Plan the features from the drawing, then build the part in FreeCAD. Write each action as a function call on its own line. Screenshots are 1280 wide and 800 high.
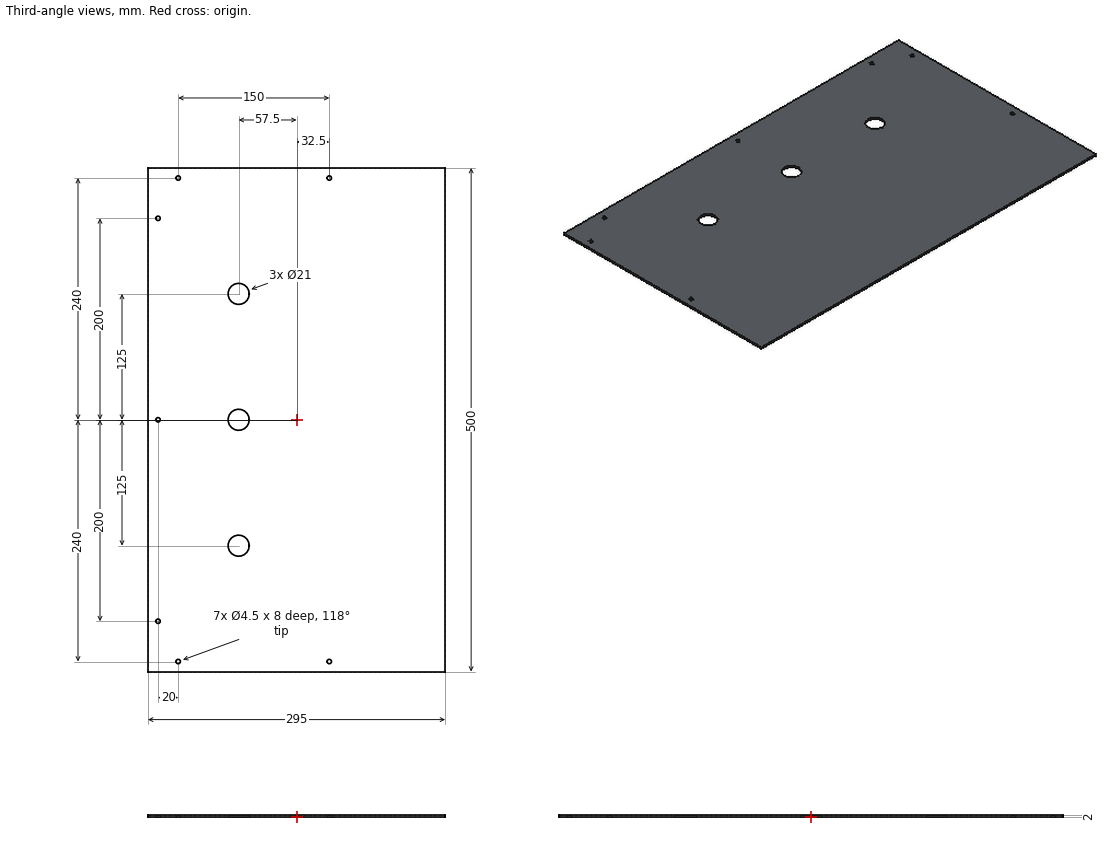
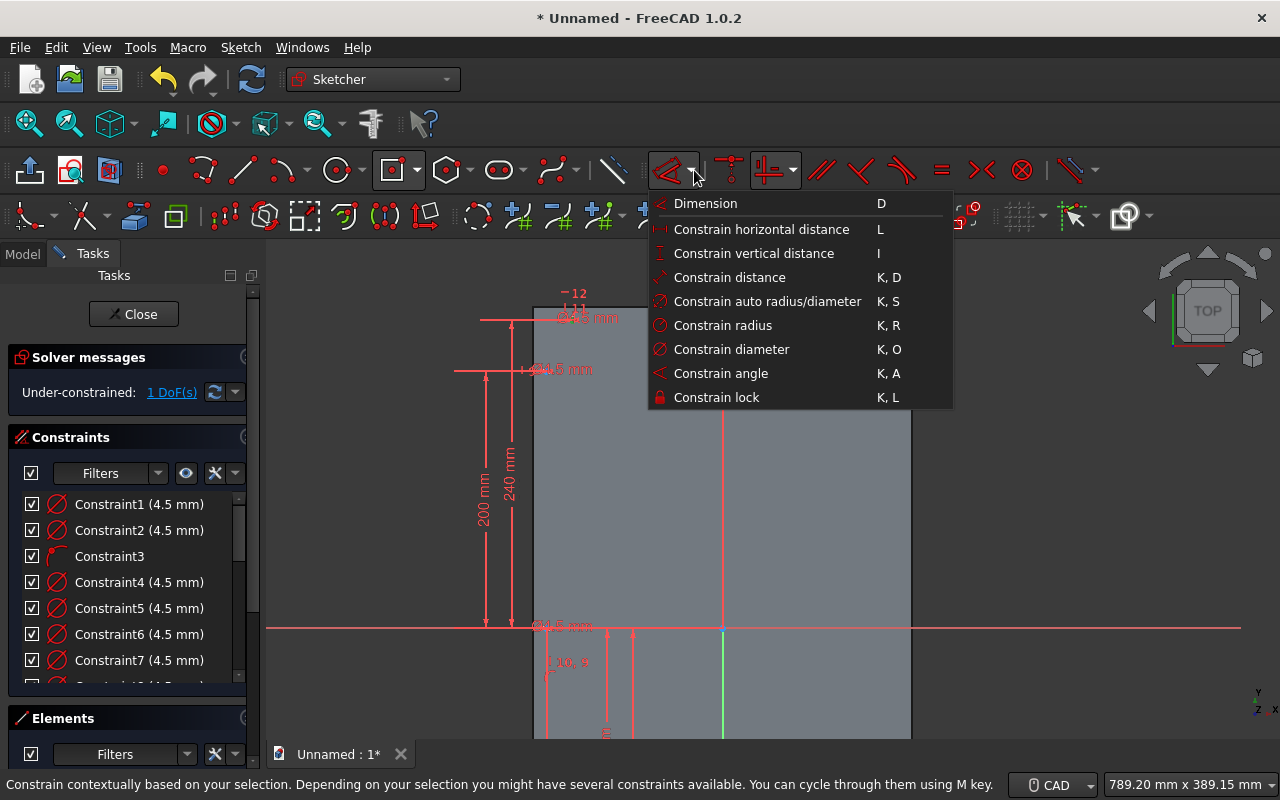
click(801, 229)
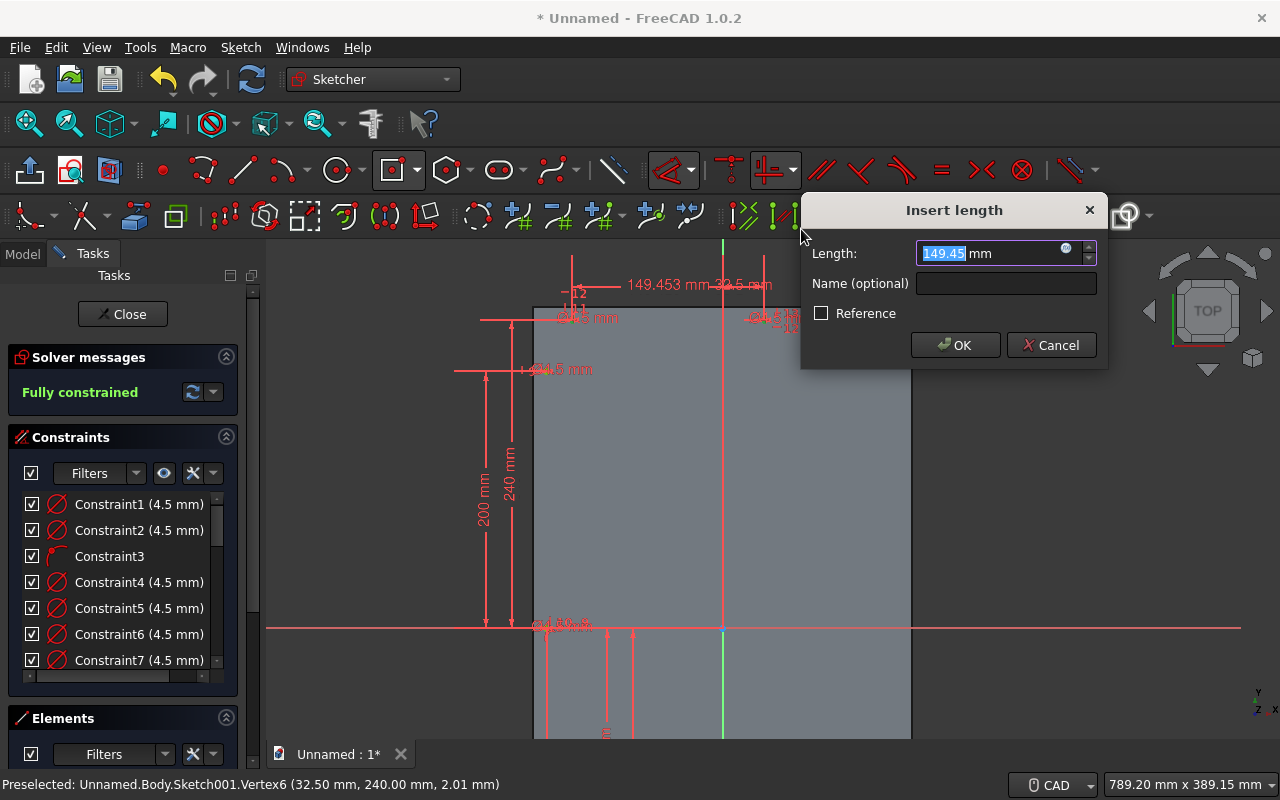
text(150)
key(Return)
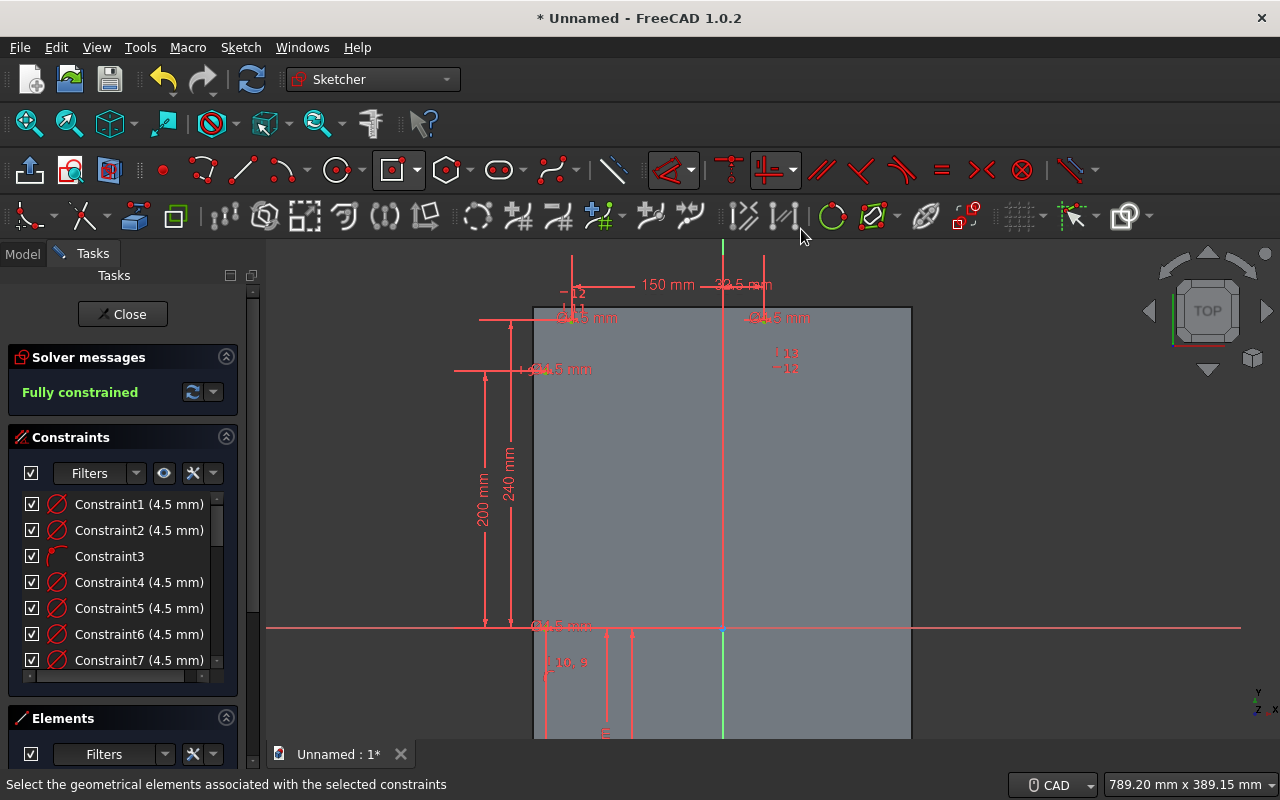
click(123, 314)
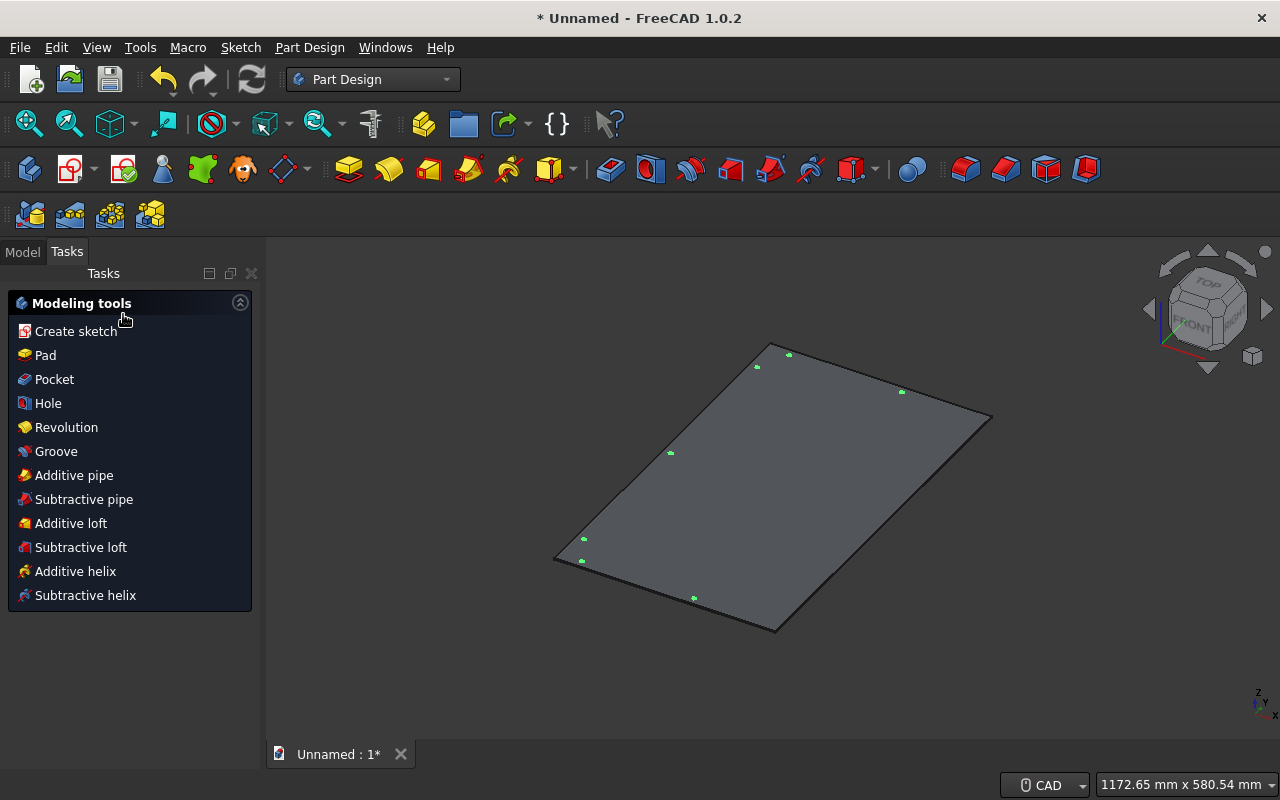
click(652, 170)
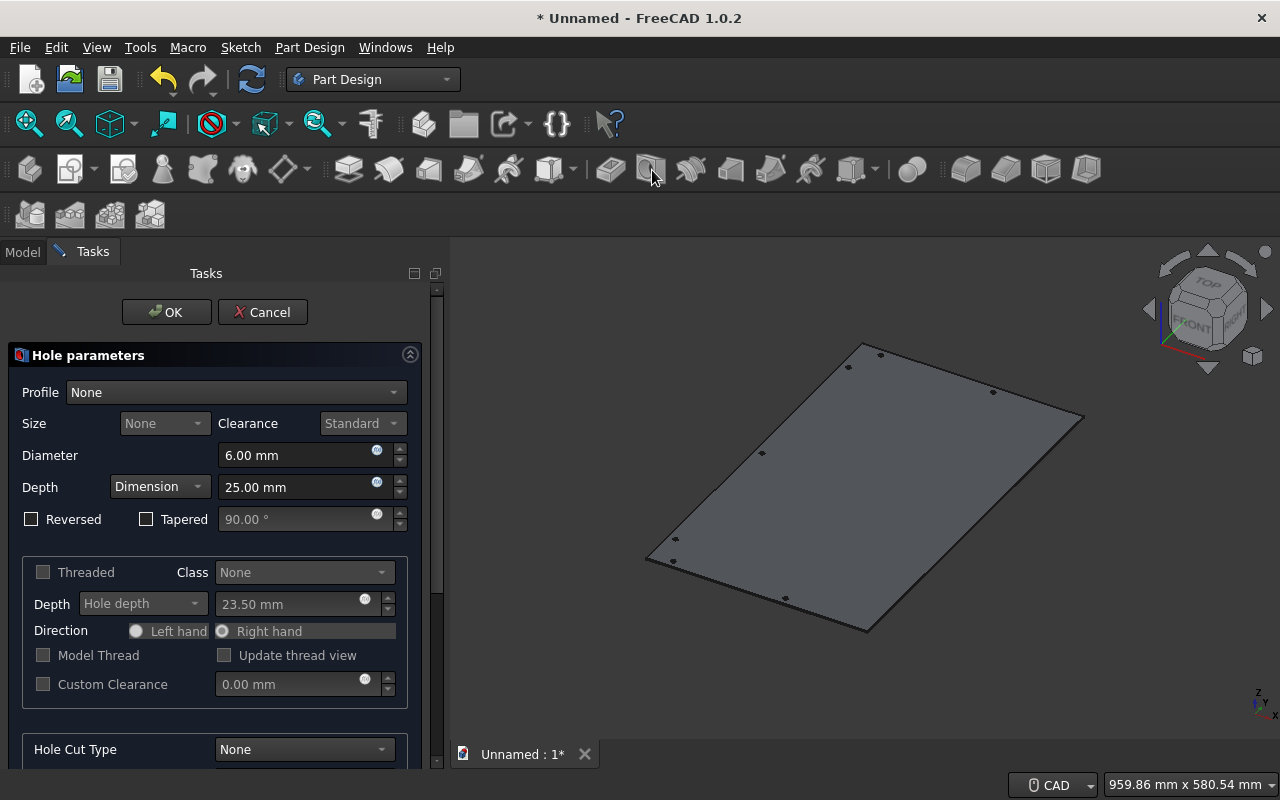
triple_click(305, 455)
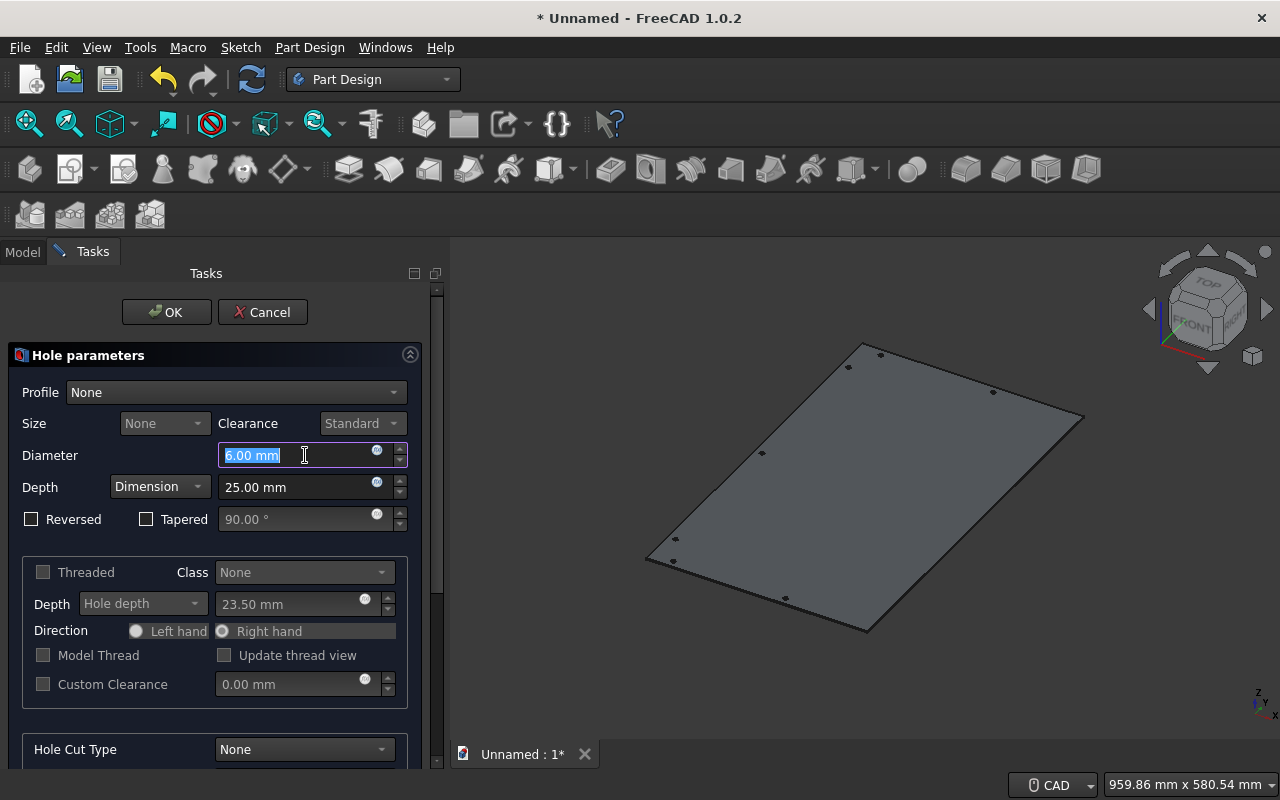
text(4.5)
key(Tab)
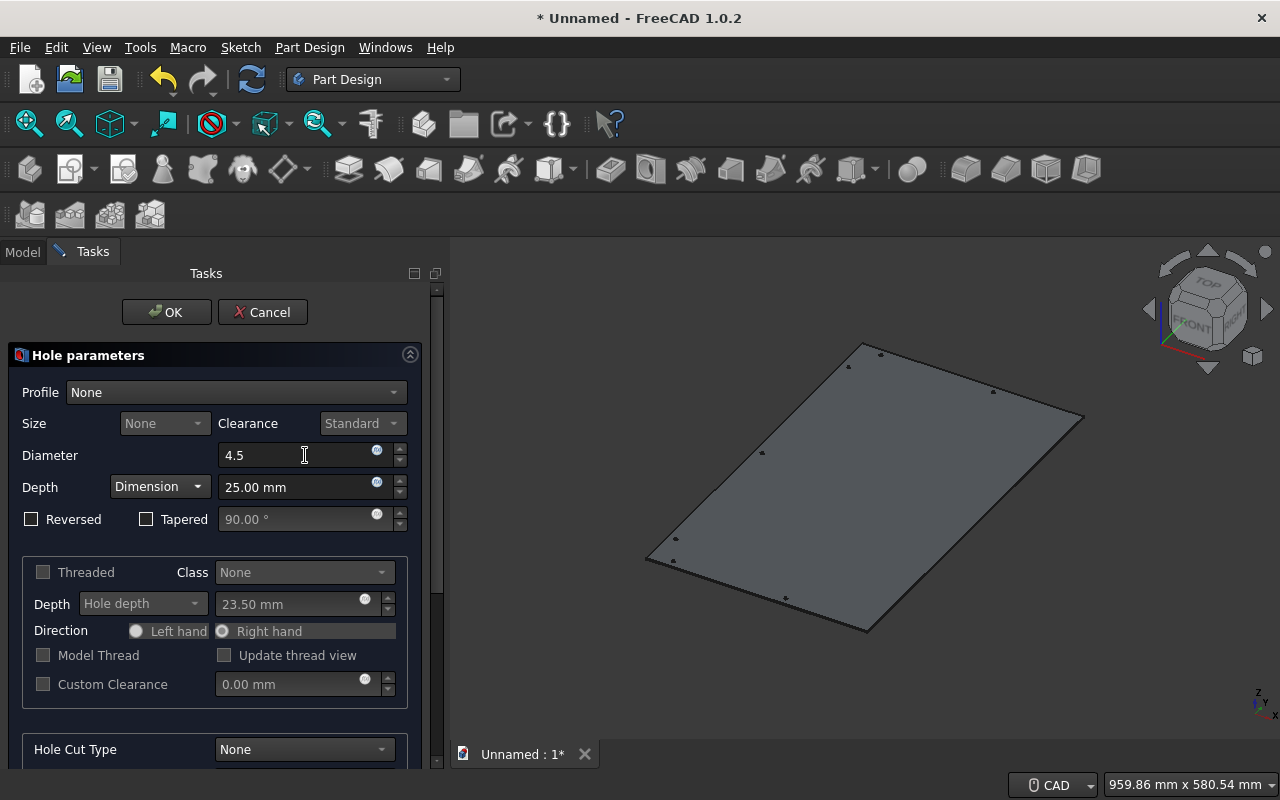
triple_click(305, 487)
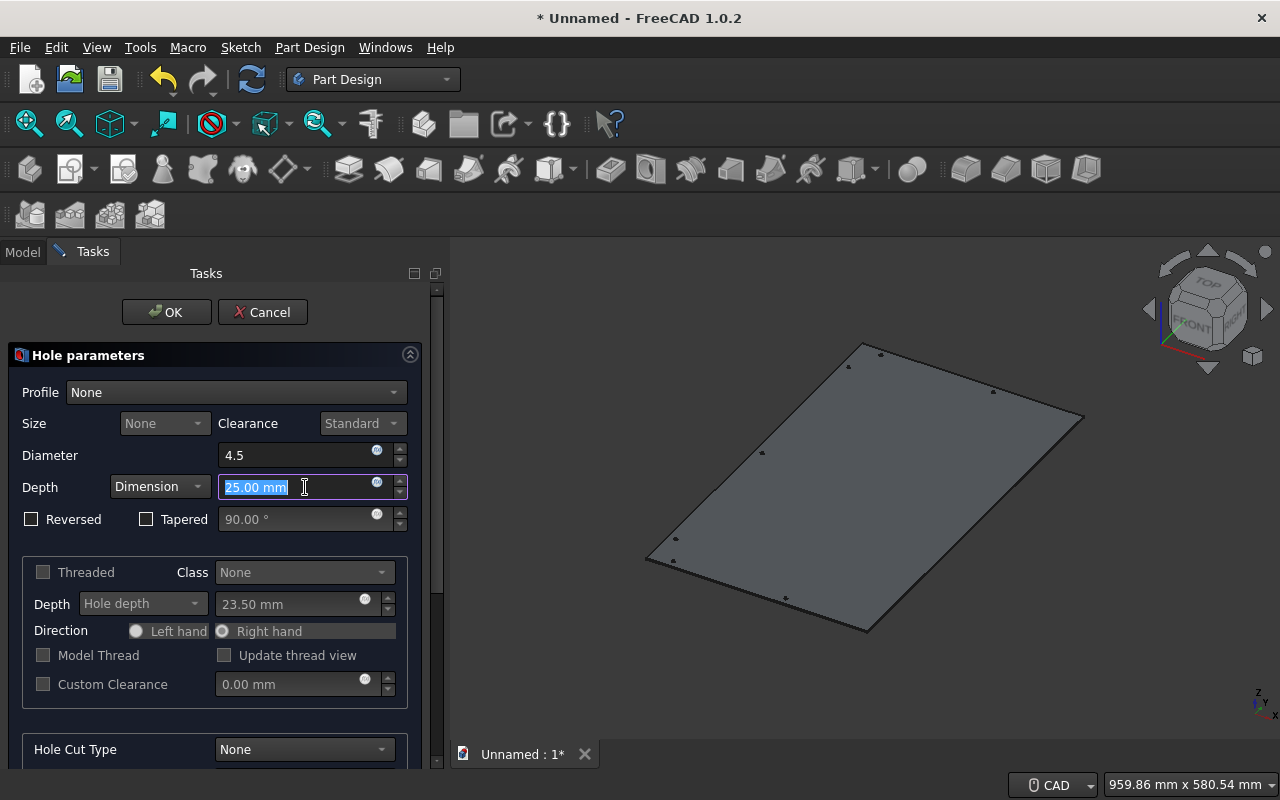
text(8)
key(Tab)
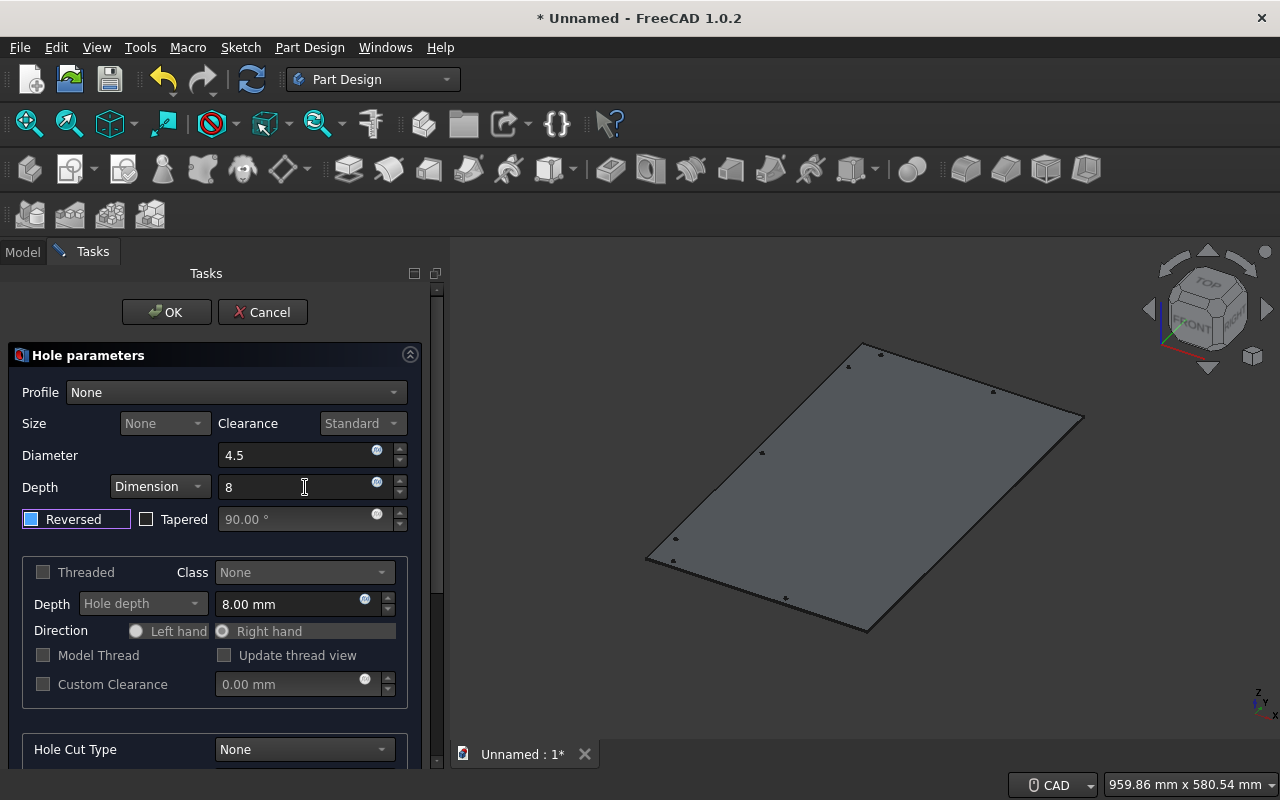
click(167, 312)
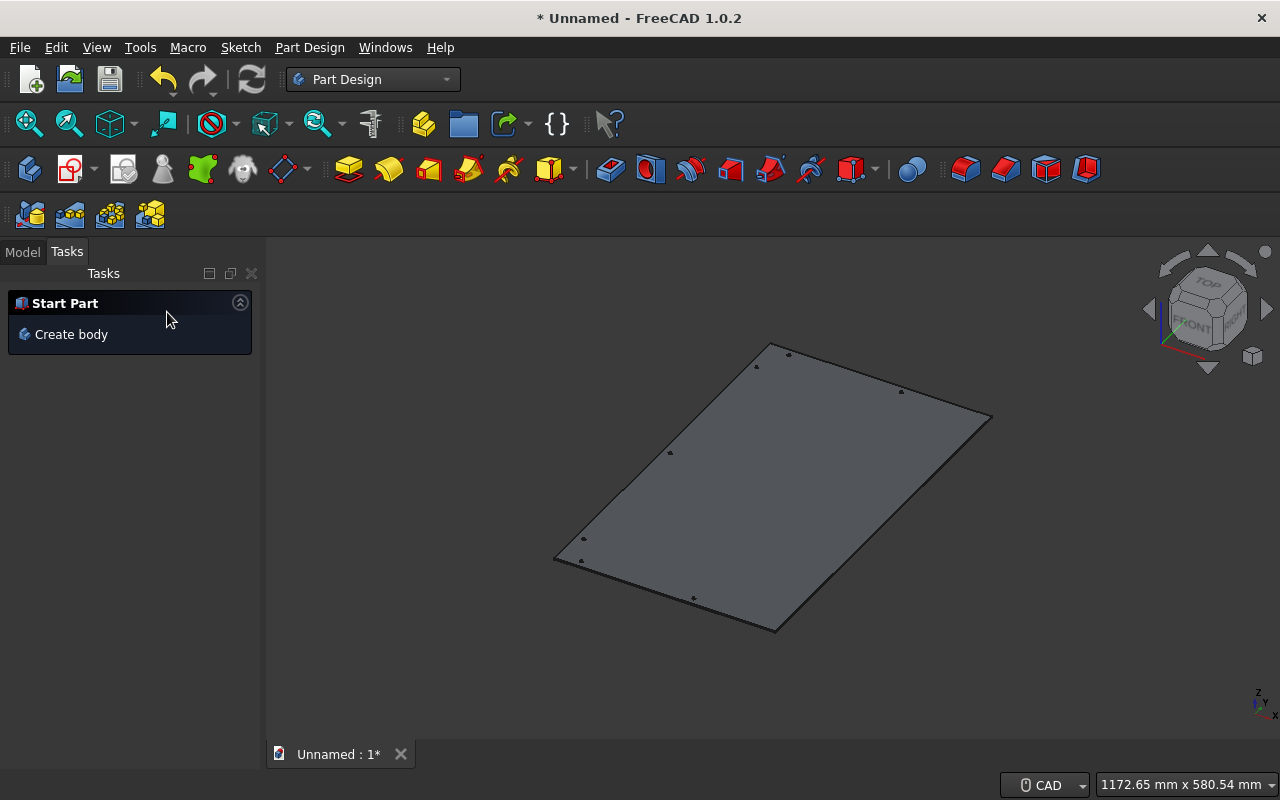
click(804, 456)